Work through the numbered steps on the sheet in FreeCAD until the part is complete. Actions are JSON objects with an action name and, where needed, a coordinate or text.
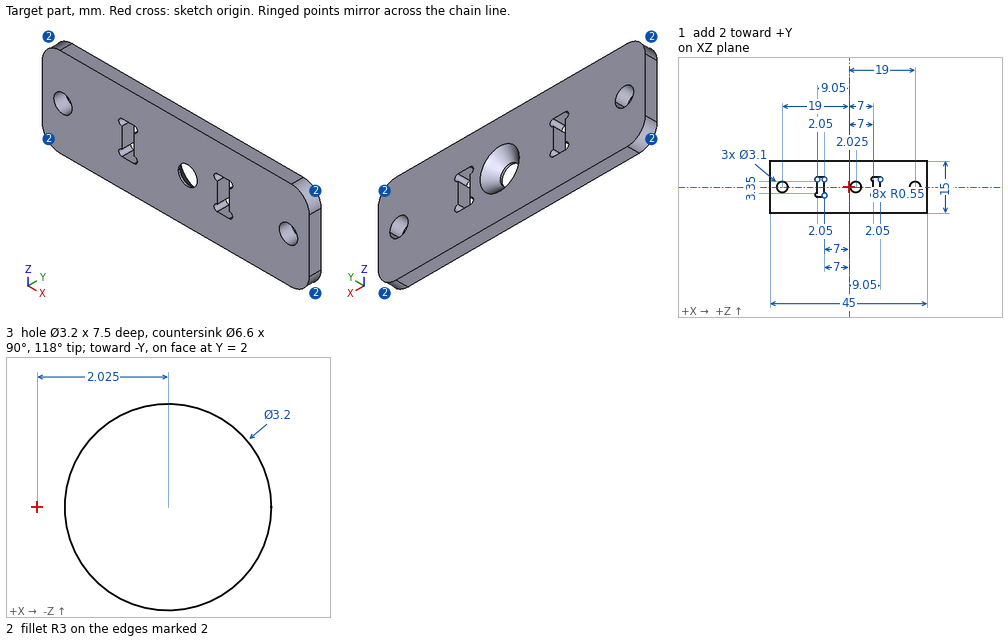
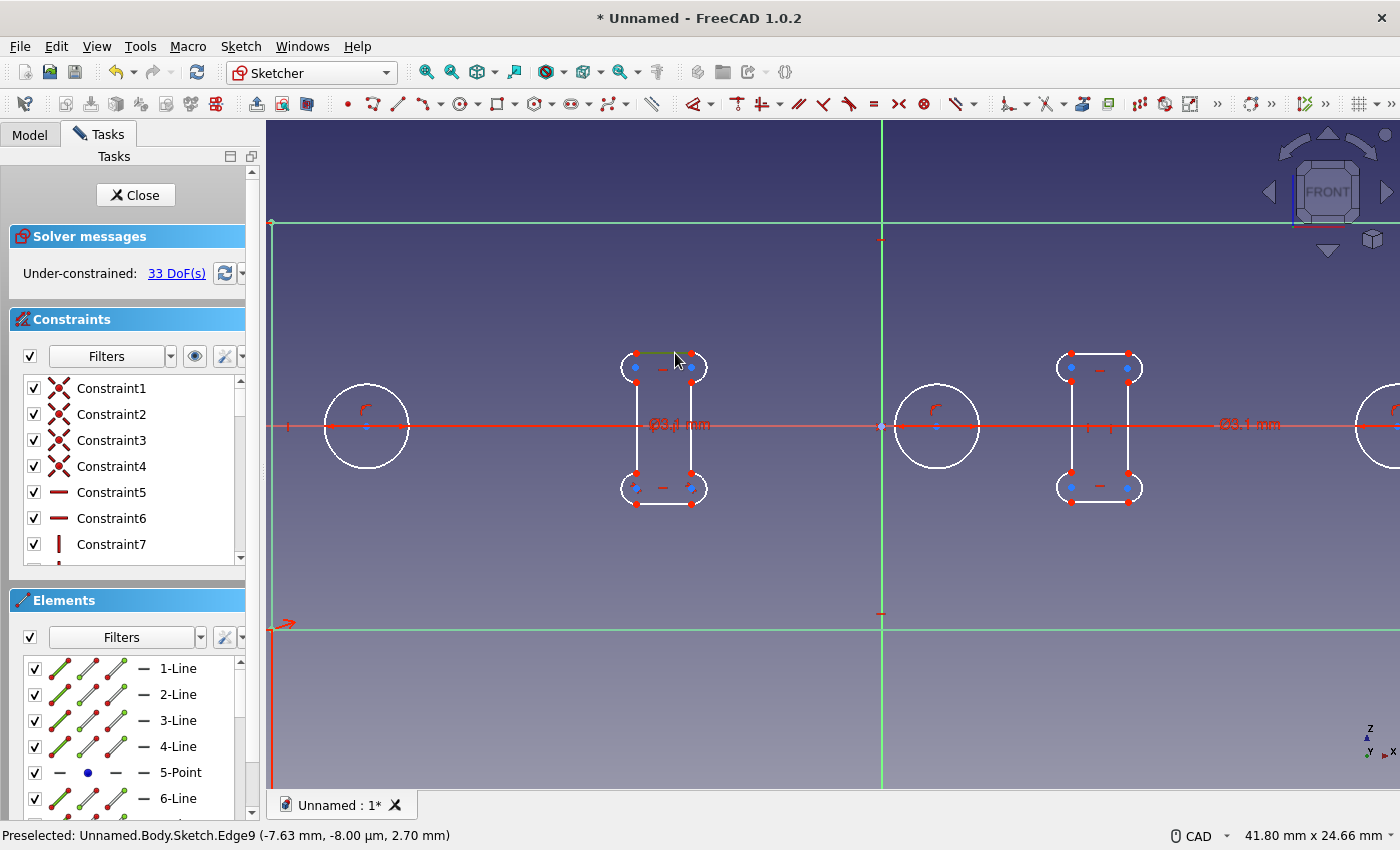
{"action": "left_click", "coordinate": [704, 376]}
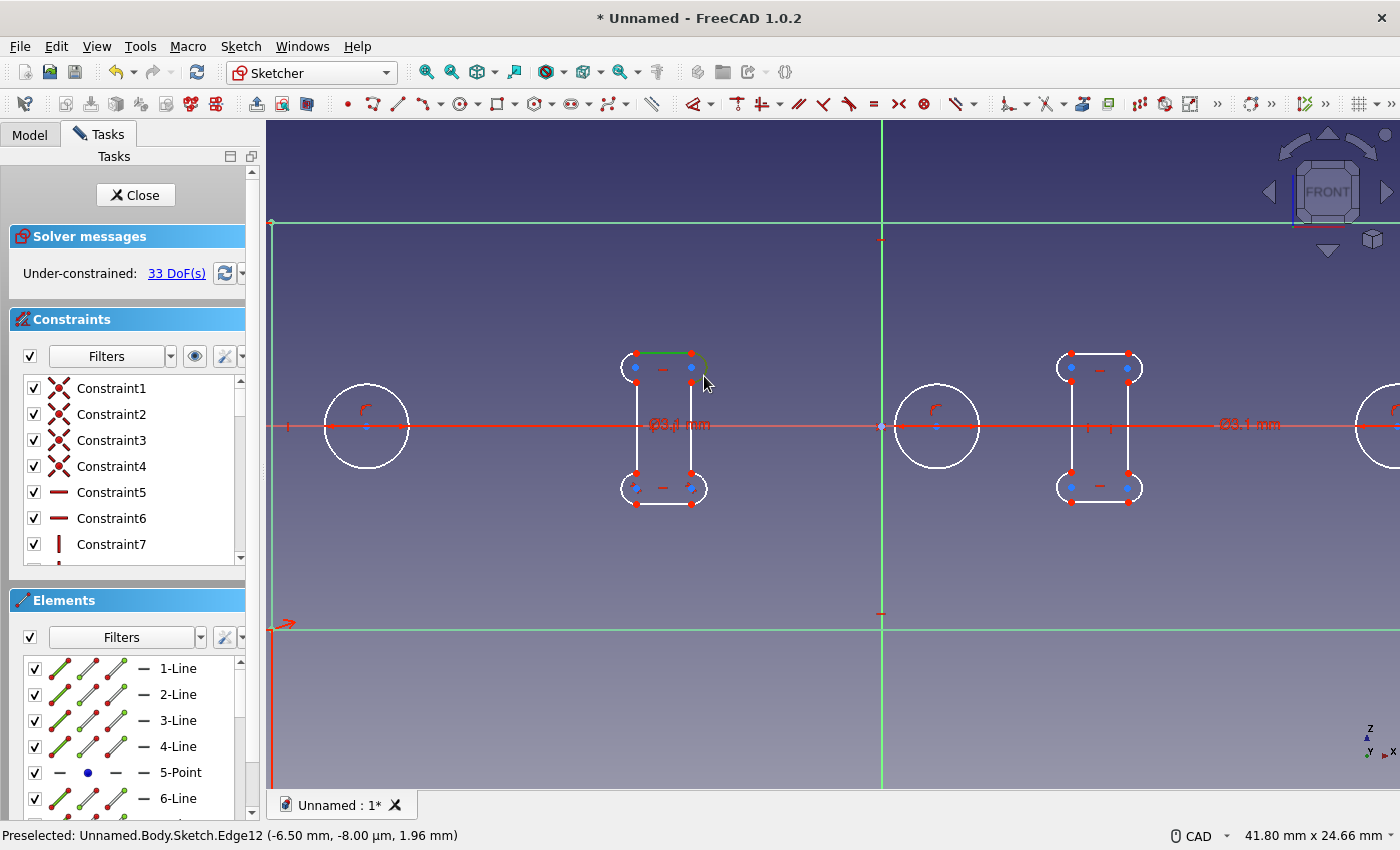
{"action": "left_click", "coordinate": [849, 104]}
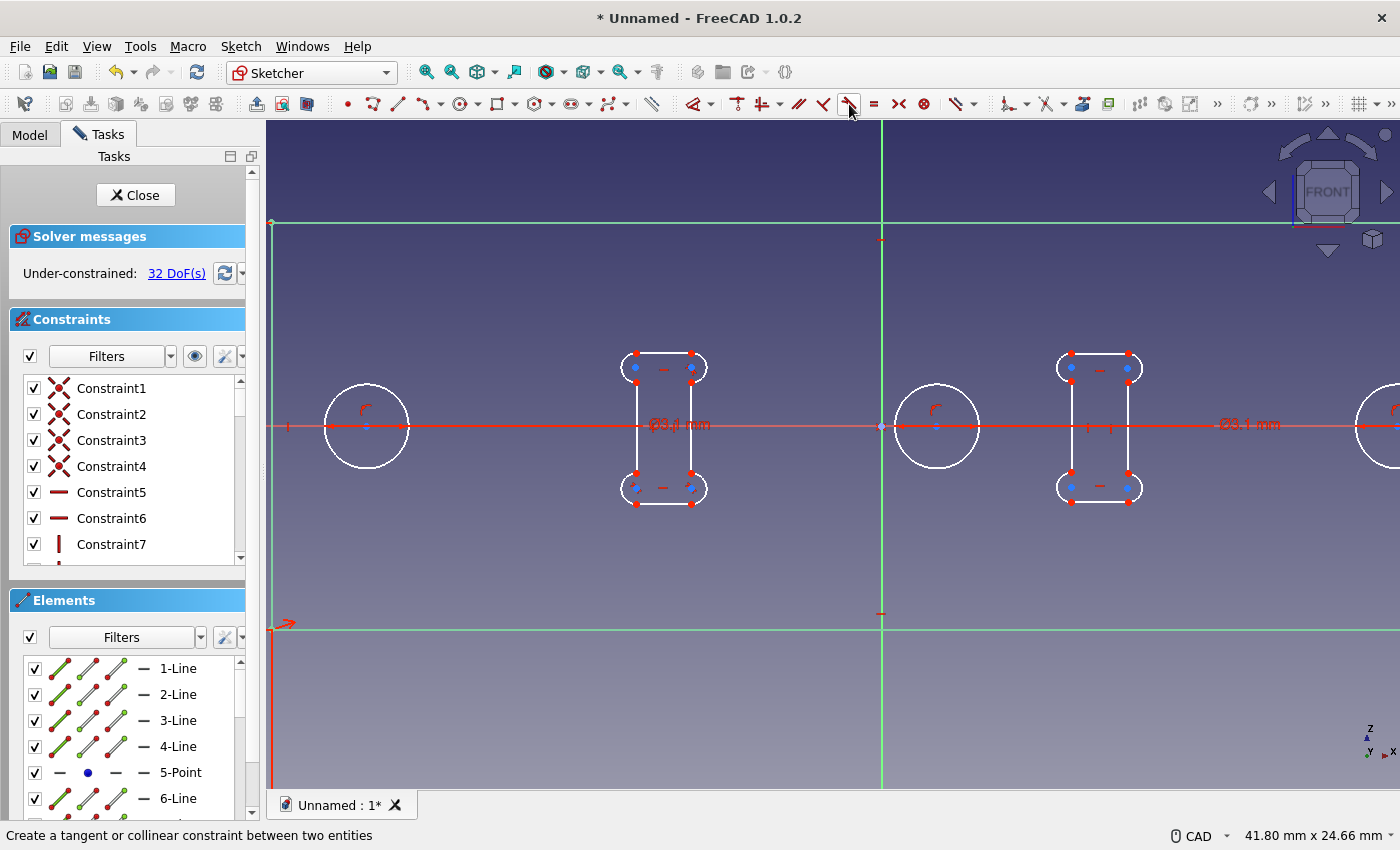
{"action": "left_click", "coordinate": [675, 353]}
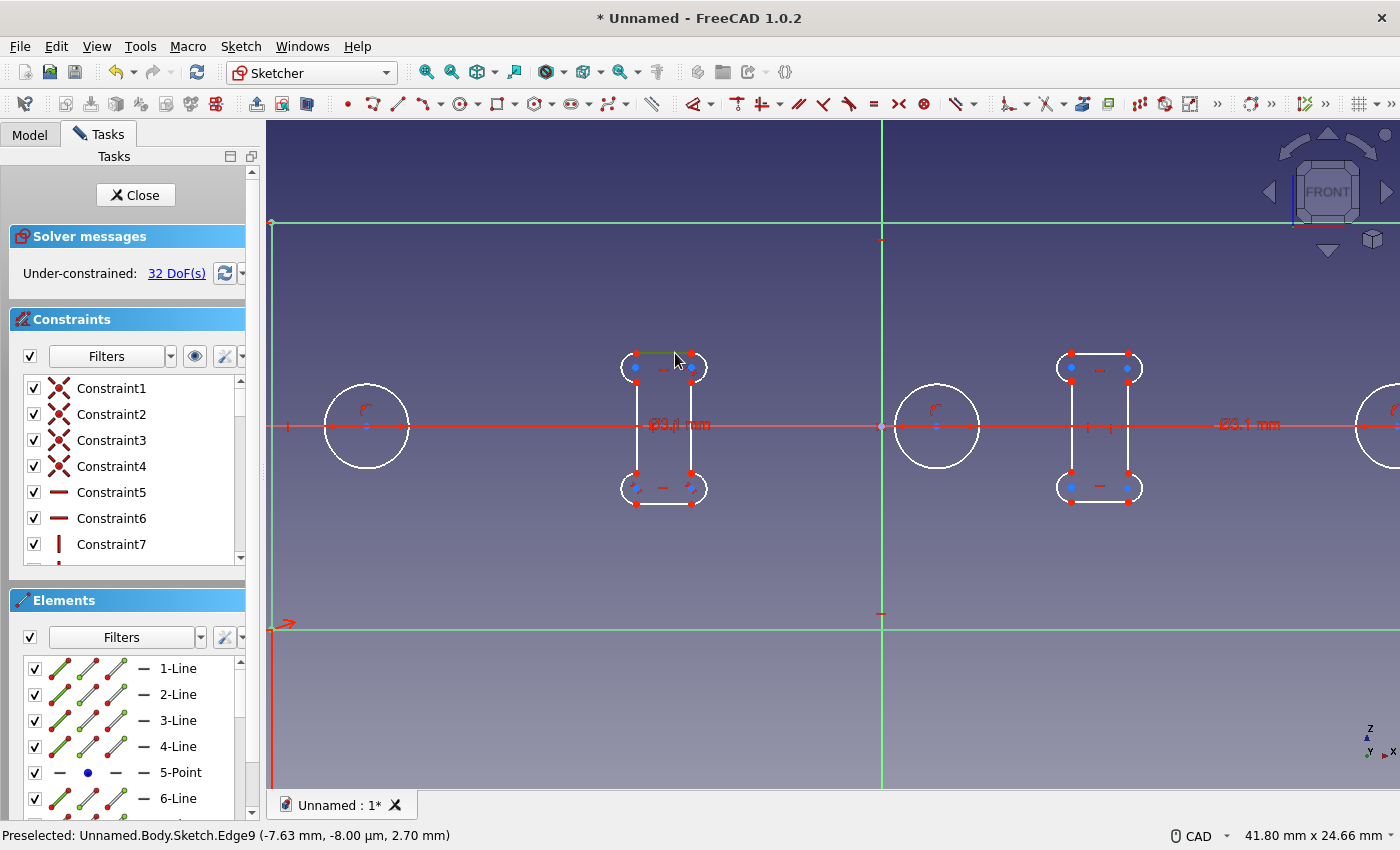
{"action": "left_click", "coordinate": [624, 359]}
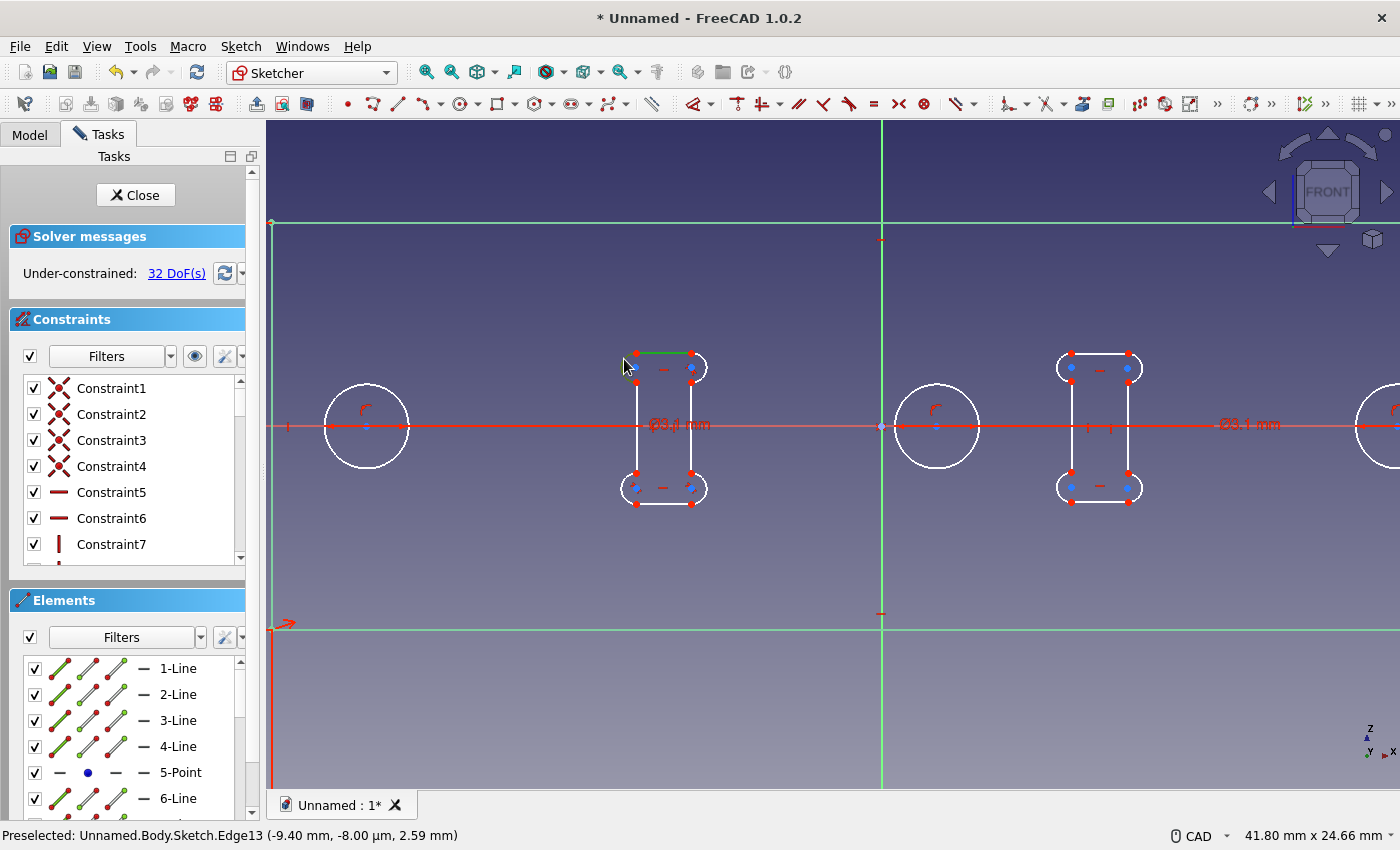
{"action": "left_click", "coordinate": [849, 104]}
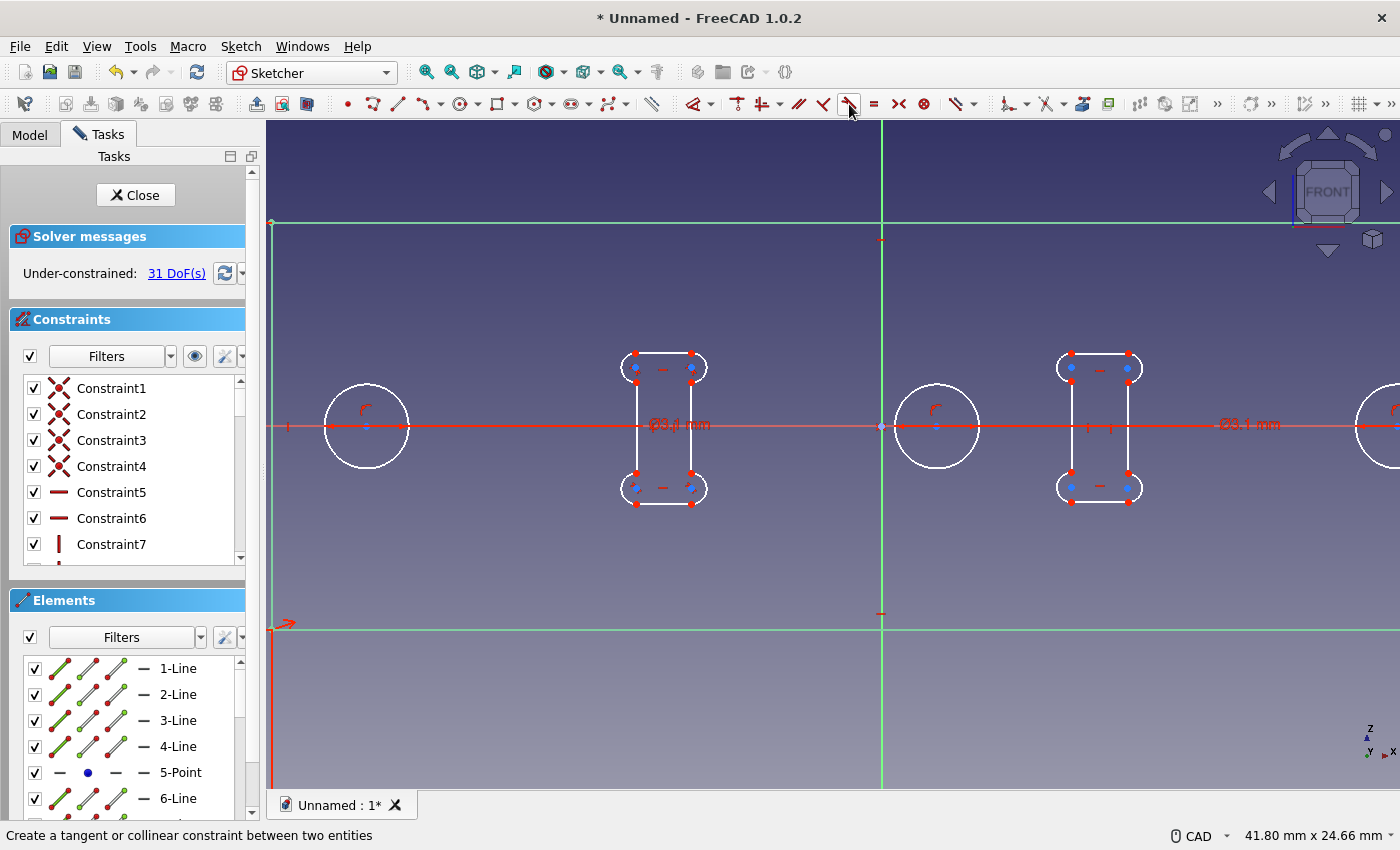
{"action": "left_click", "coordinate": [1089, 502]}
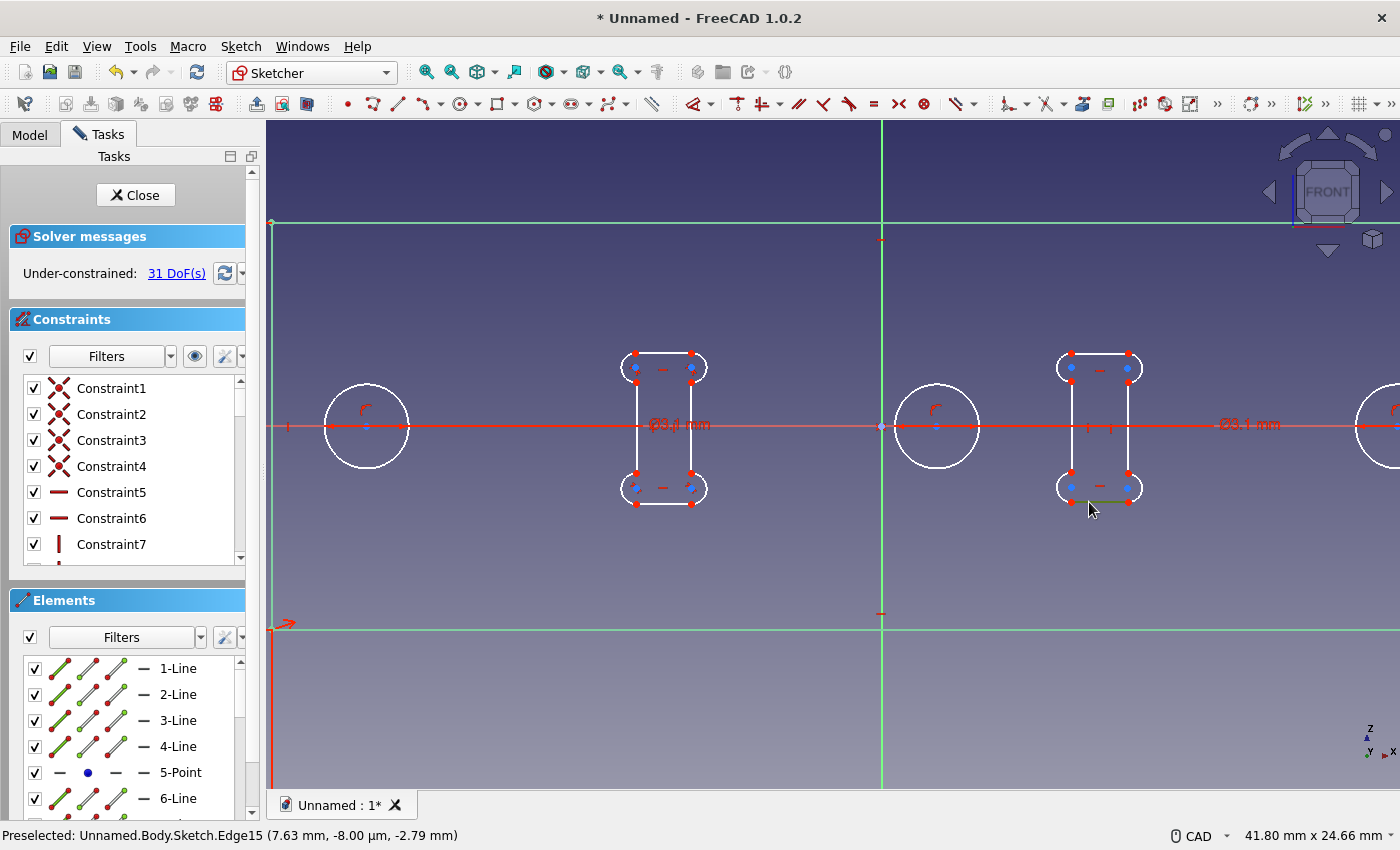
{"action": "left_click", "coordinate": [1060, 479]}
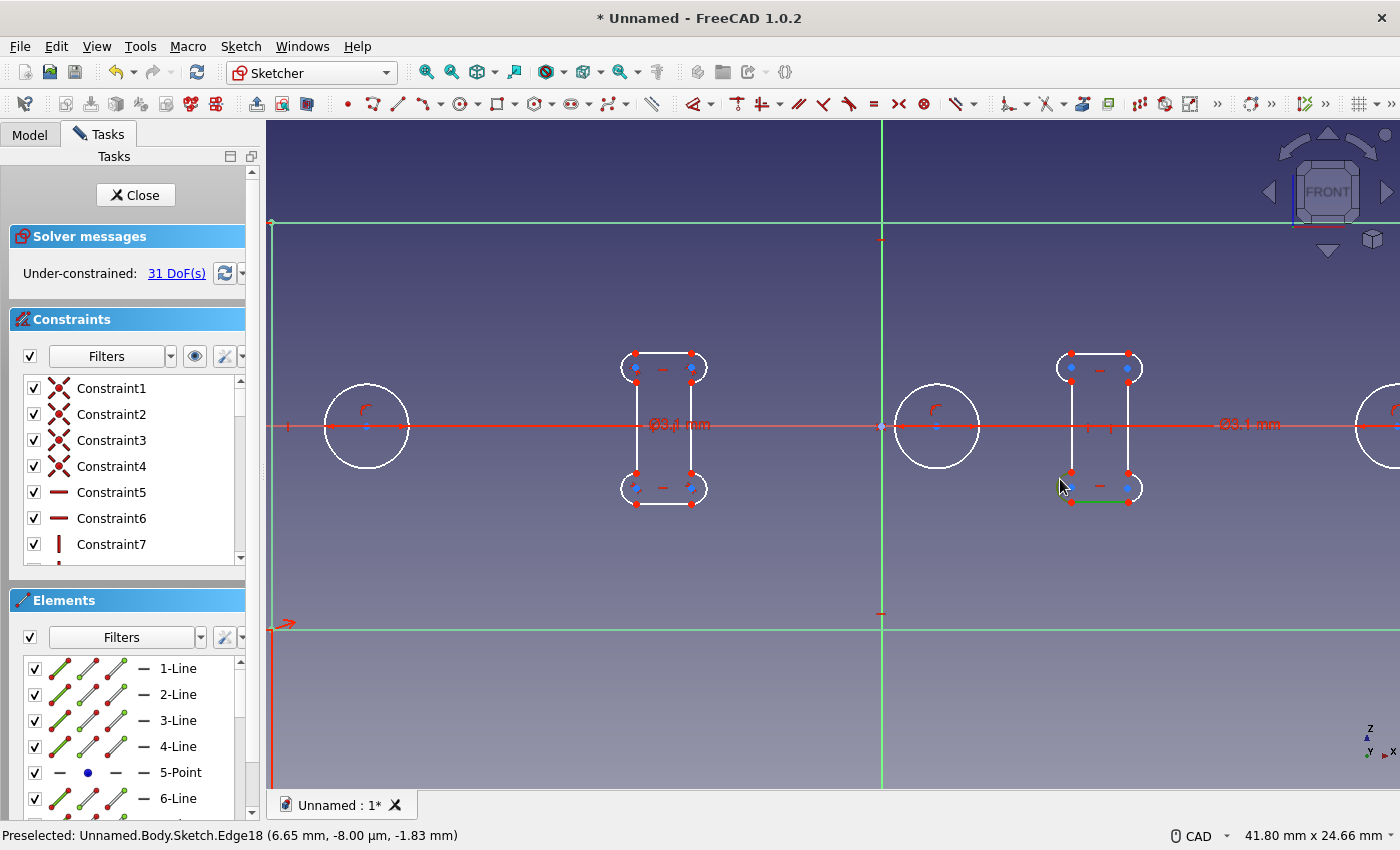
{"action": "left_click", "coordinate": [849, 104]}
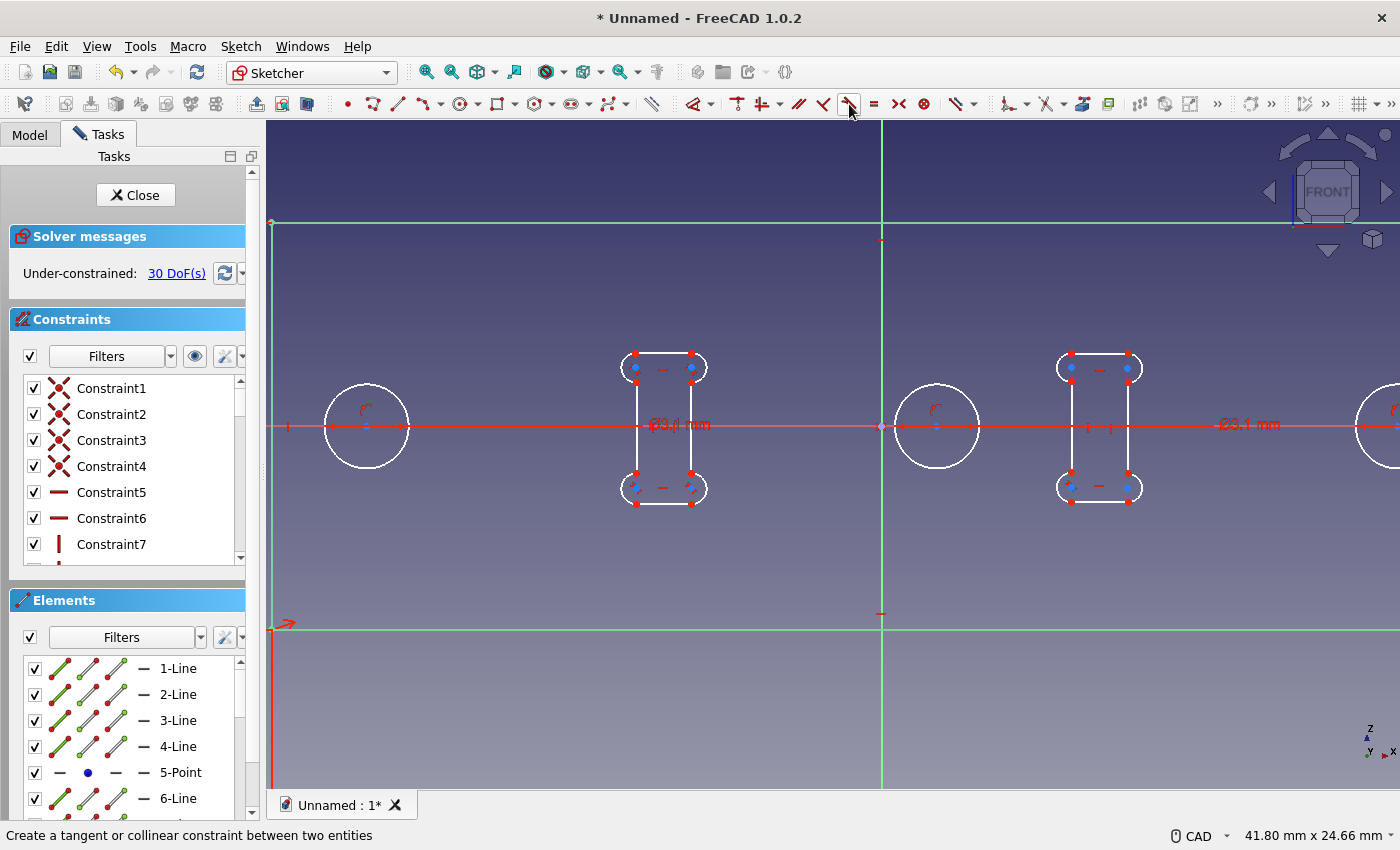
{"action": "left_click", "coordinate": [1089, 502]}